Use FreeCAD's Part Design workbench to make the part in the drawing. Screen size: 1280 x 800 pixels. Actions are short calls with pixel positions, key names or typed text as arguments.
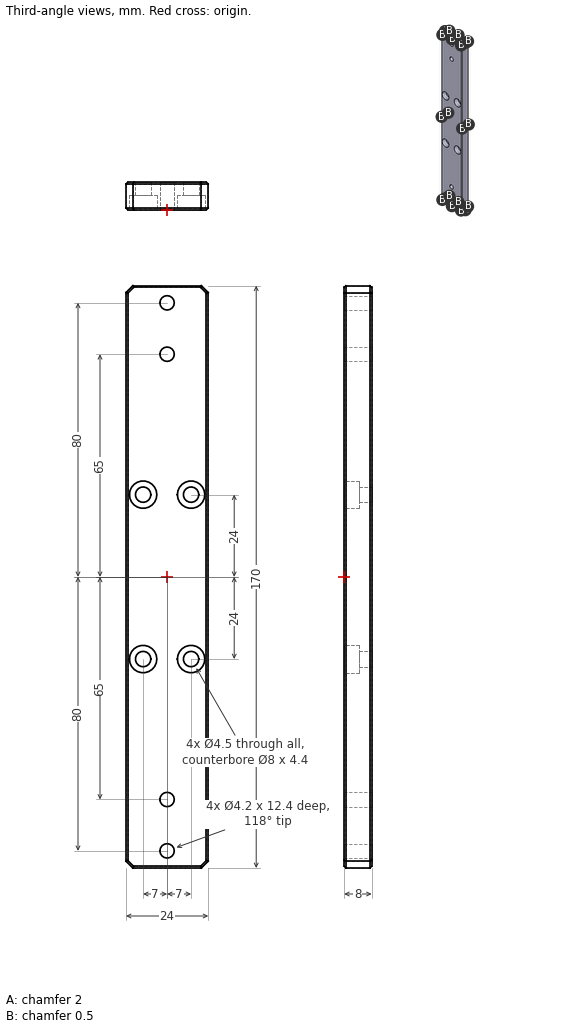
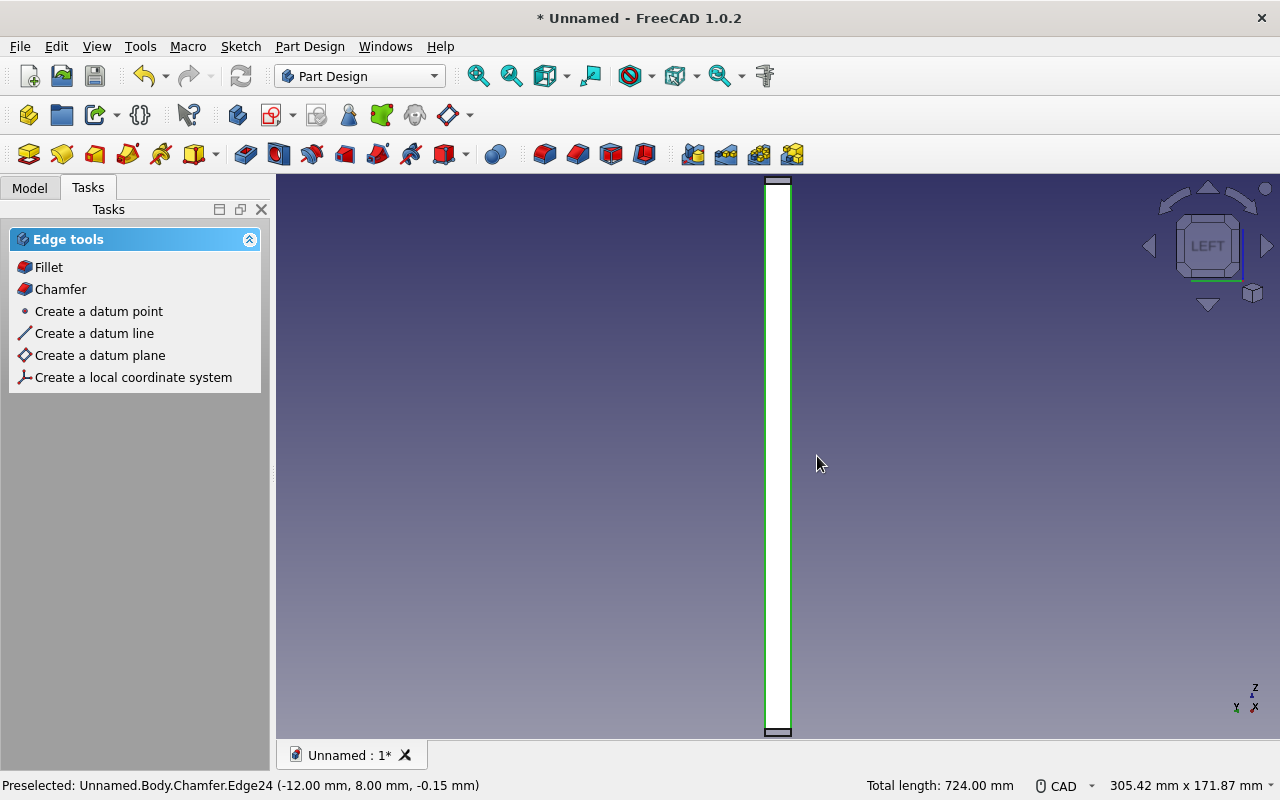
key(v)
key(3)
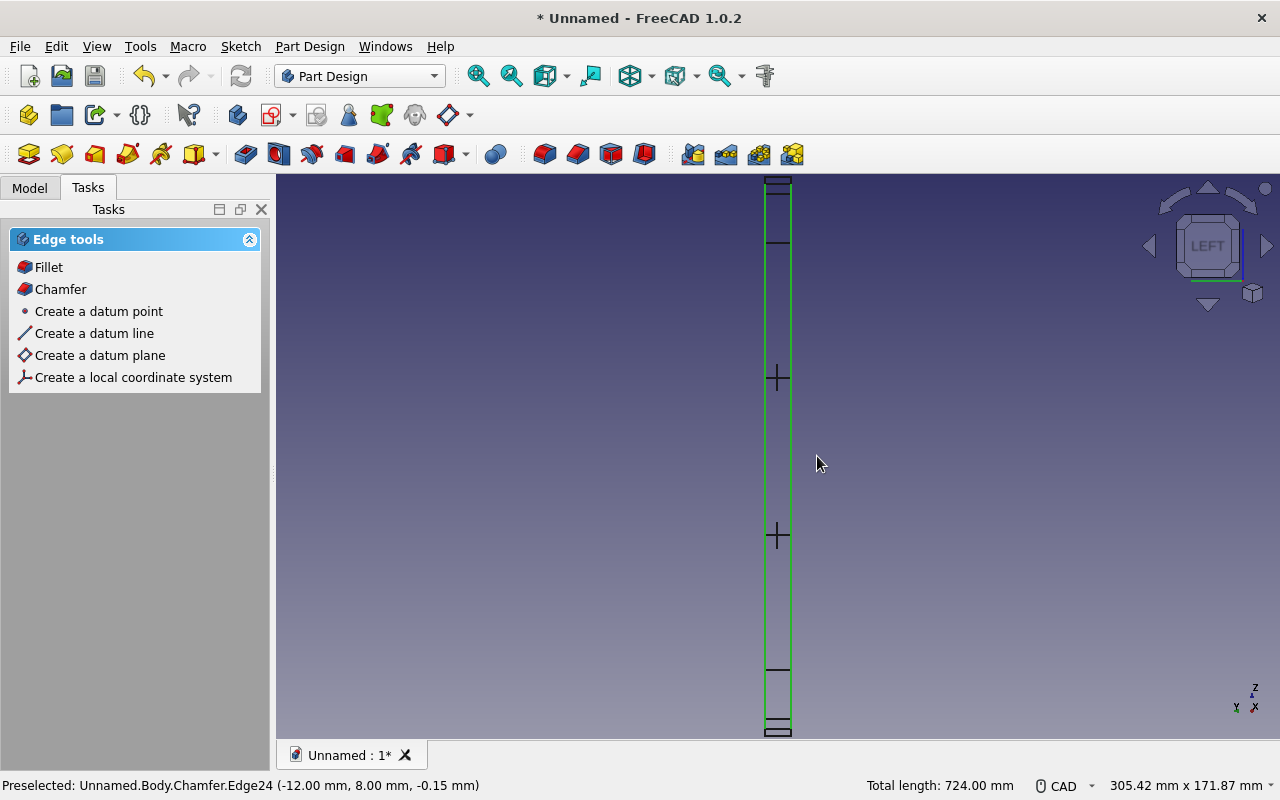
key(0)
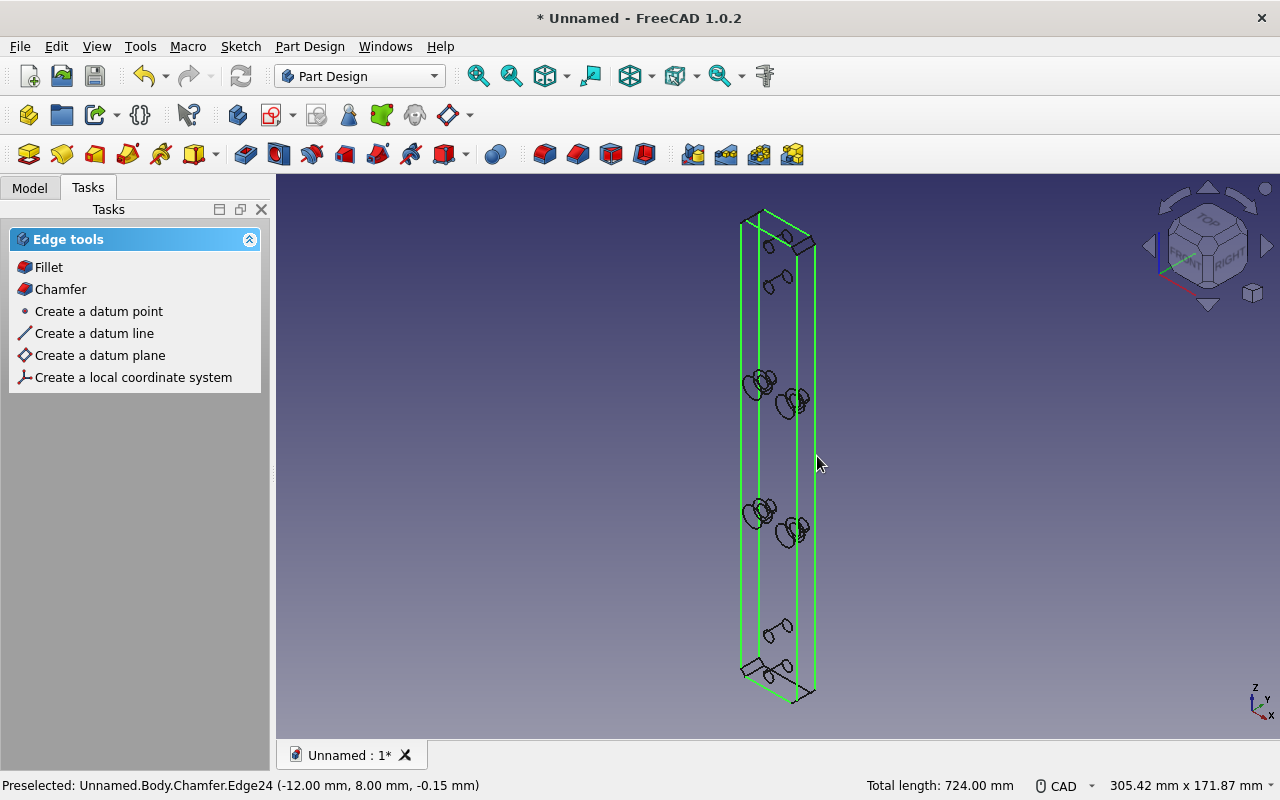
click(787, 678, ctrl)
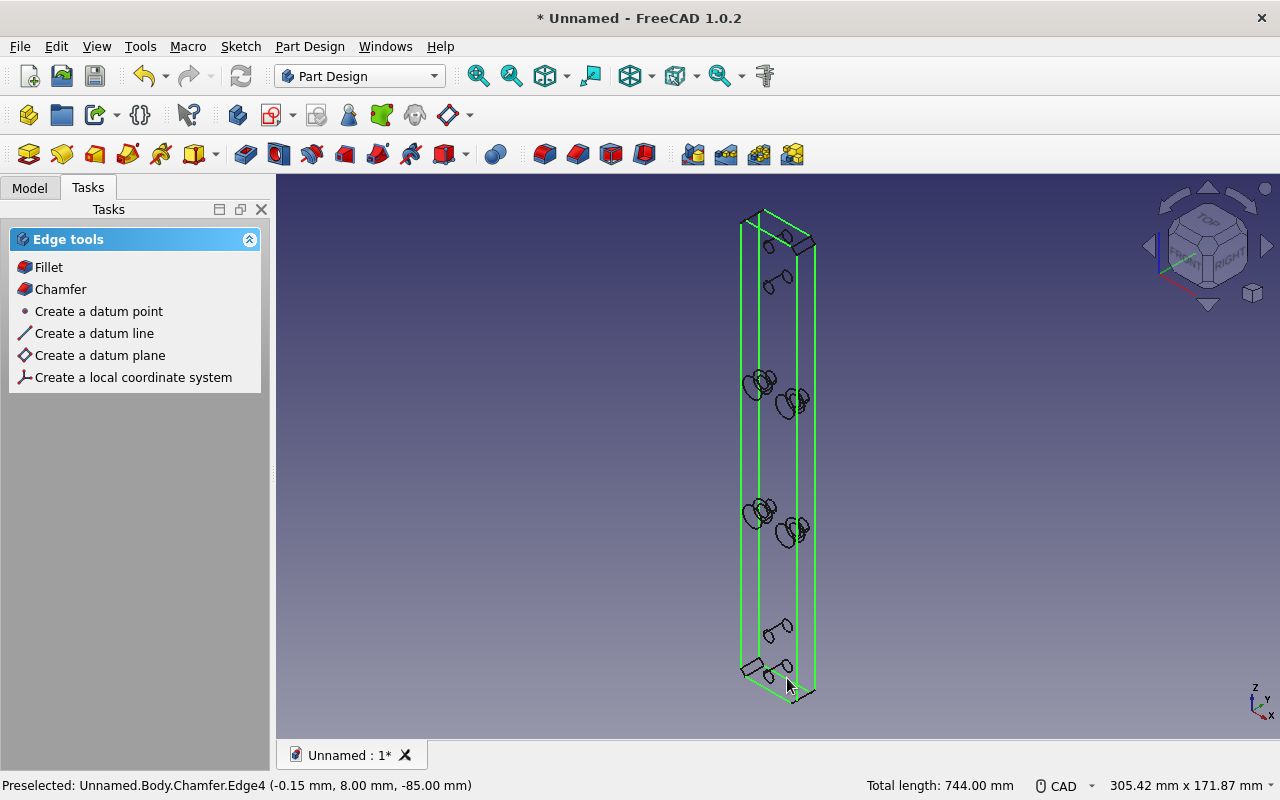
scroll(794, 250, up, 8)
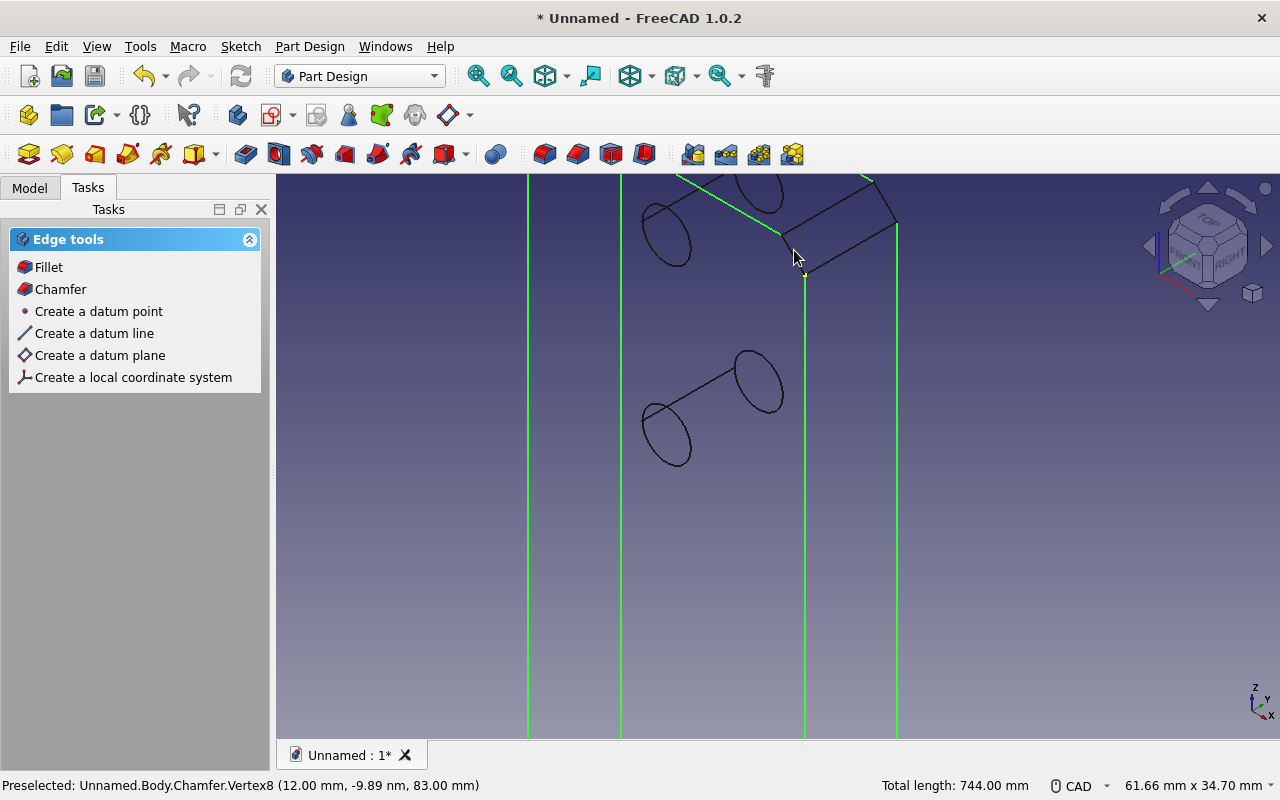
click(793, 254, ctrl)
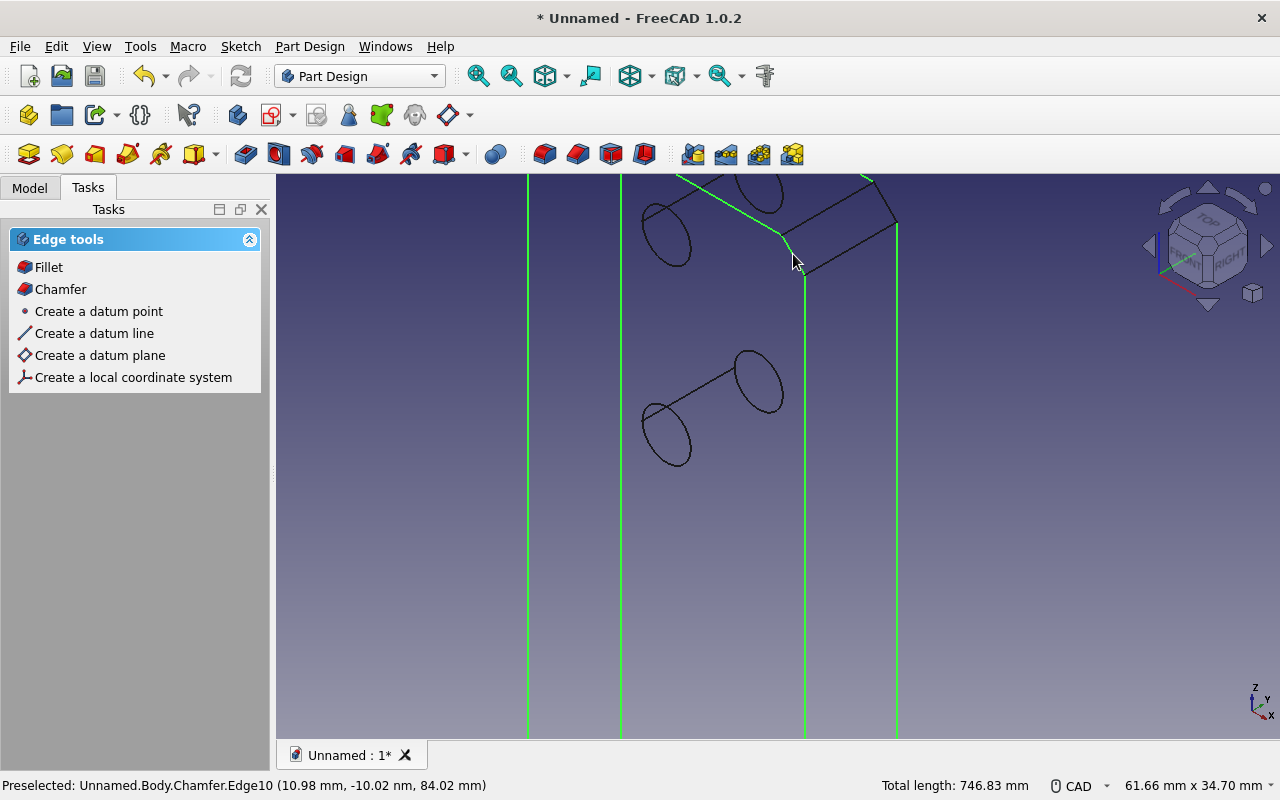
click(888, 205, ctrl)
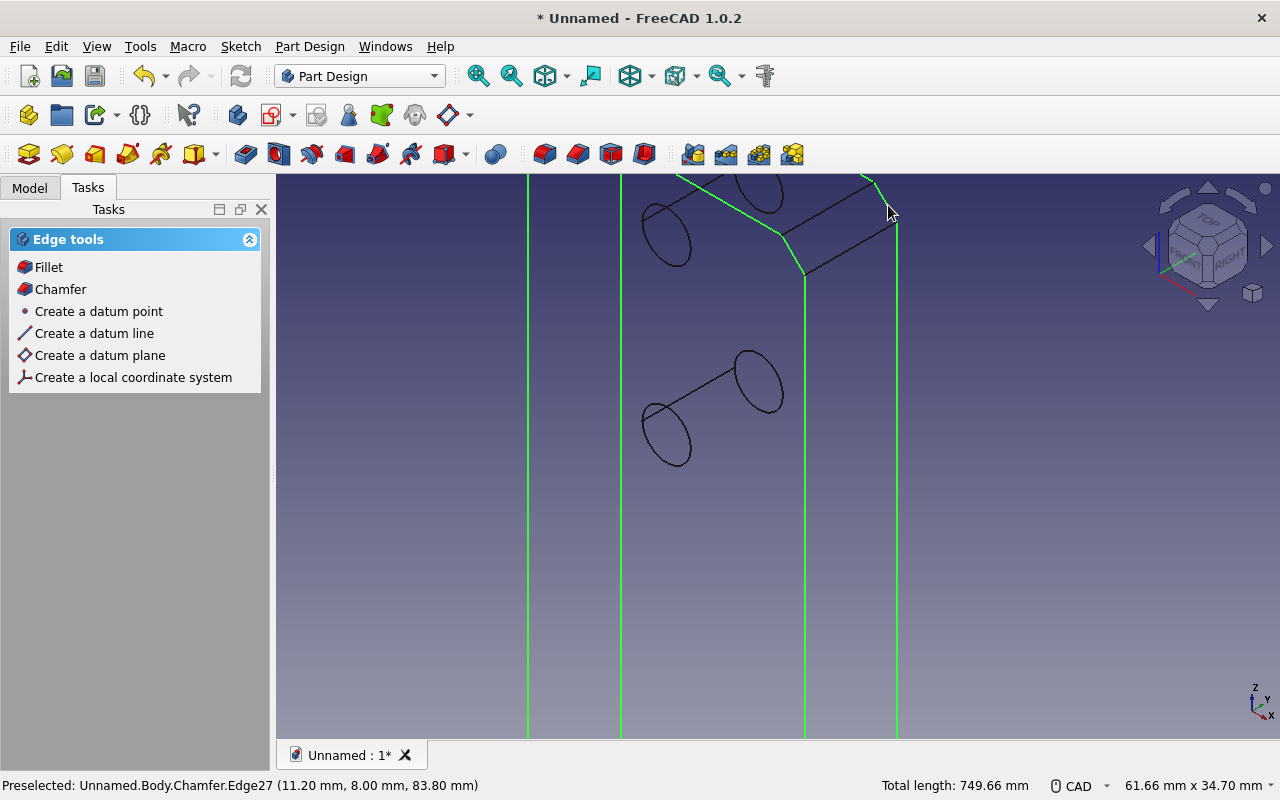
key(v)
key(f)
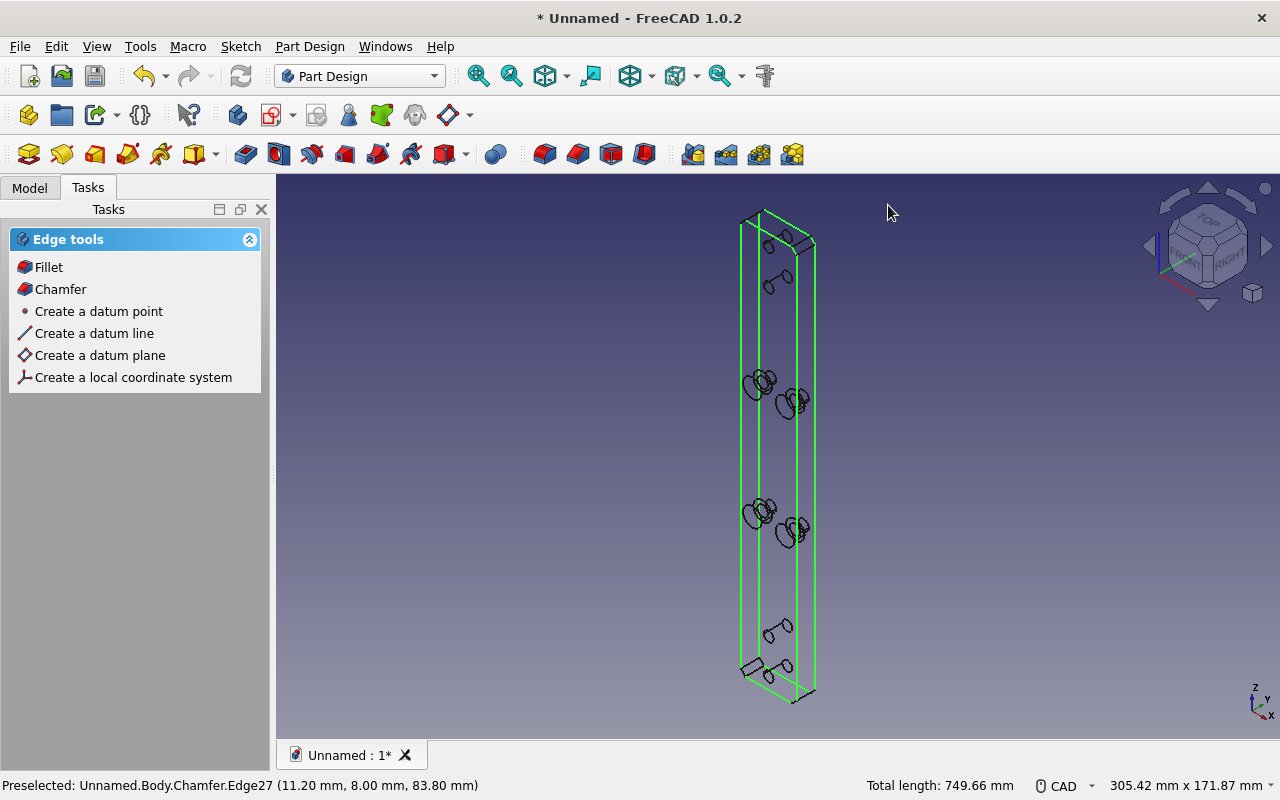
key(2)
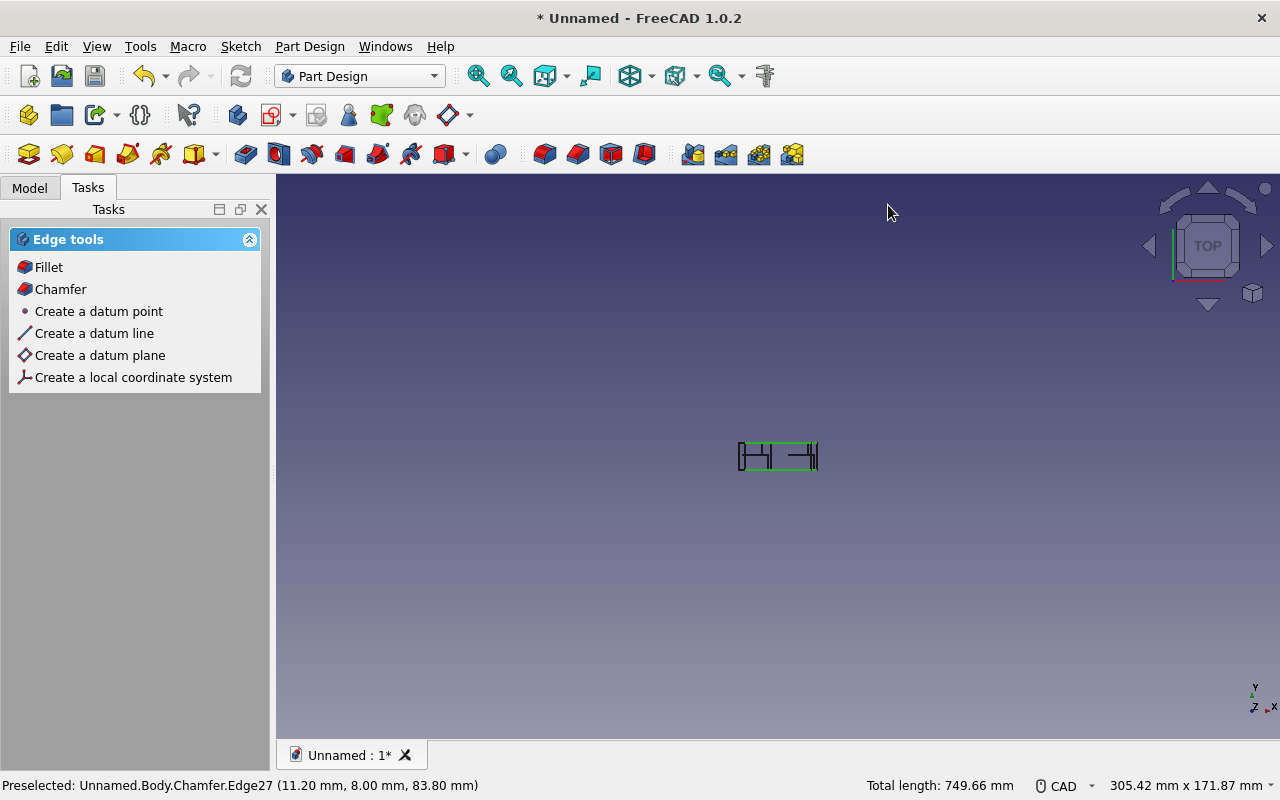
click(479, 76)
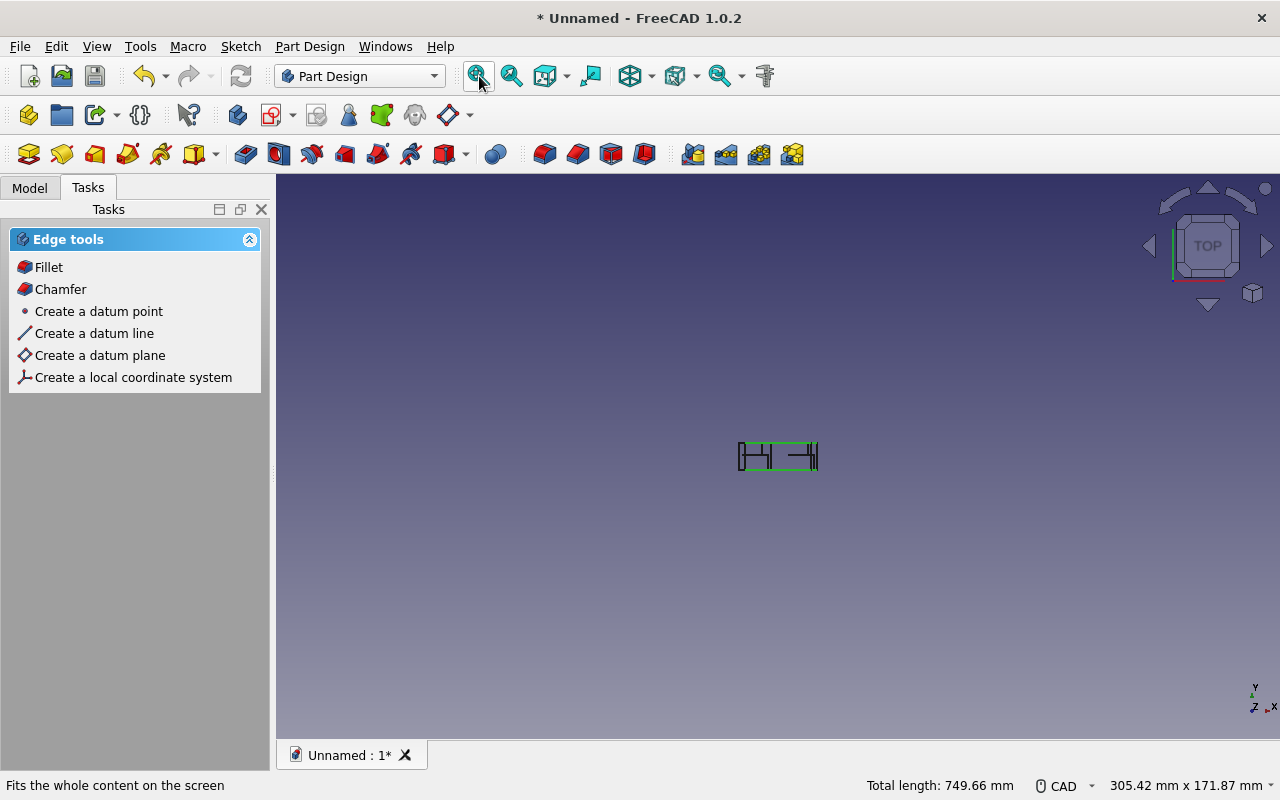
scroll(742, 469, up, 8)